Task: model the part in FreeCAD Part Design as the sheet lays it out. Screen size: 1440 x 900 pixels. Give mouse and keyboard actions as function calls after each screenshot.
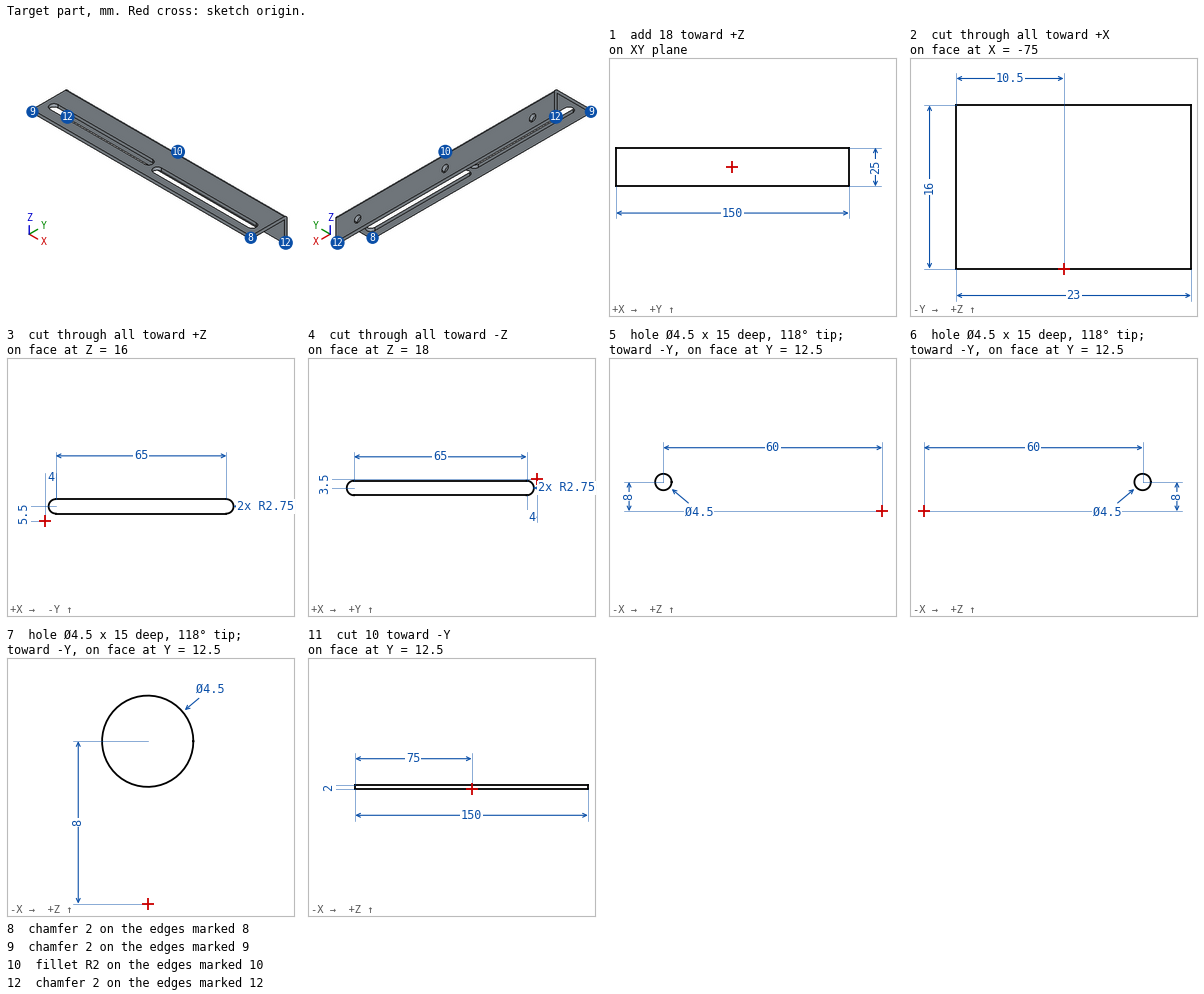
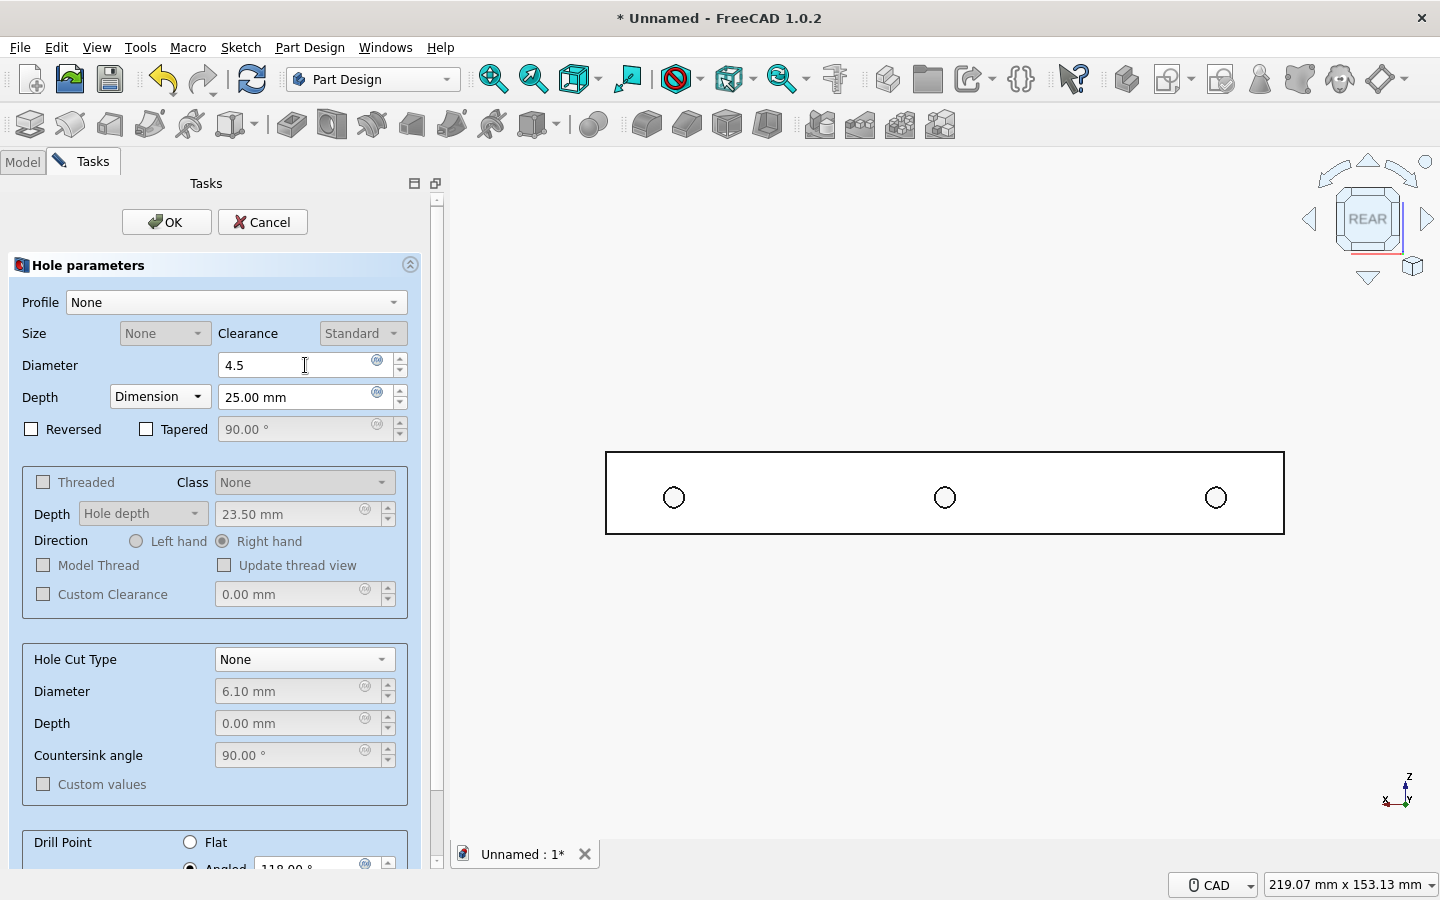
triple_click(305, 397)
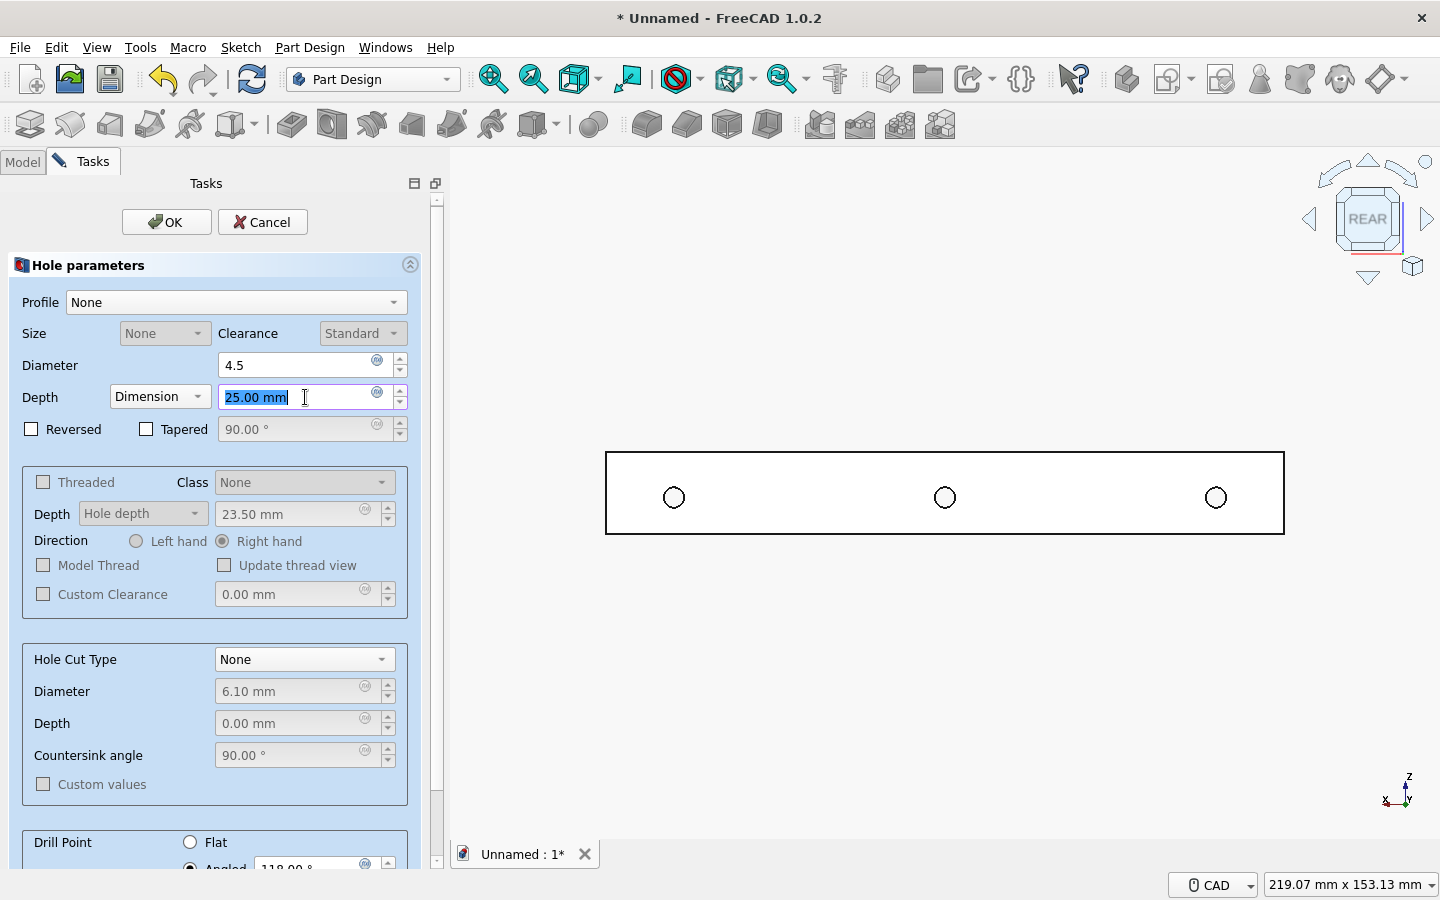
text(15)
key(Tab)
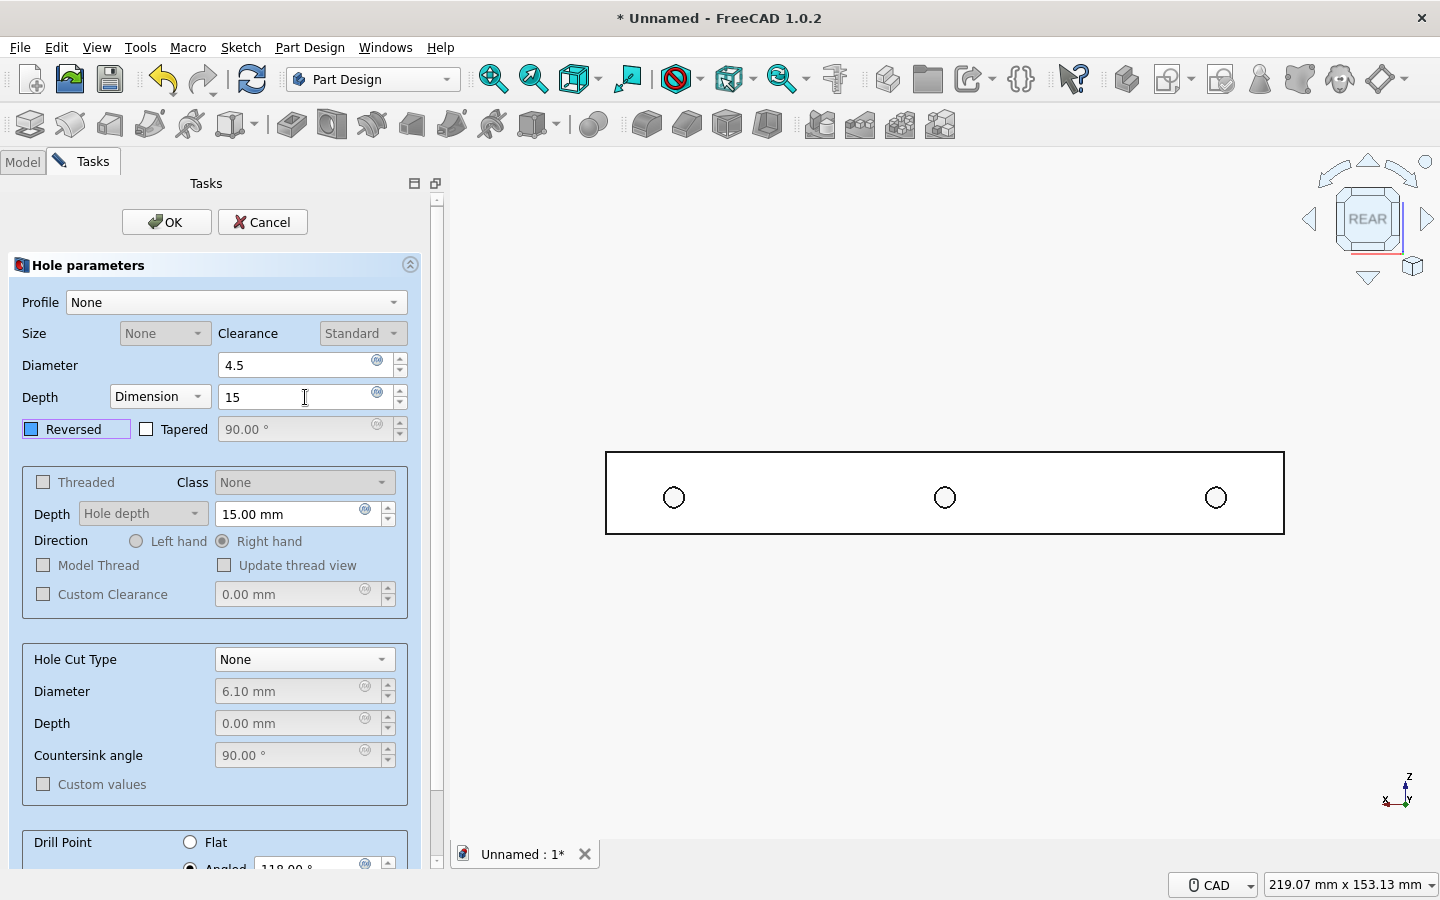
click(167, 222)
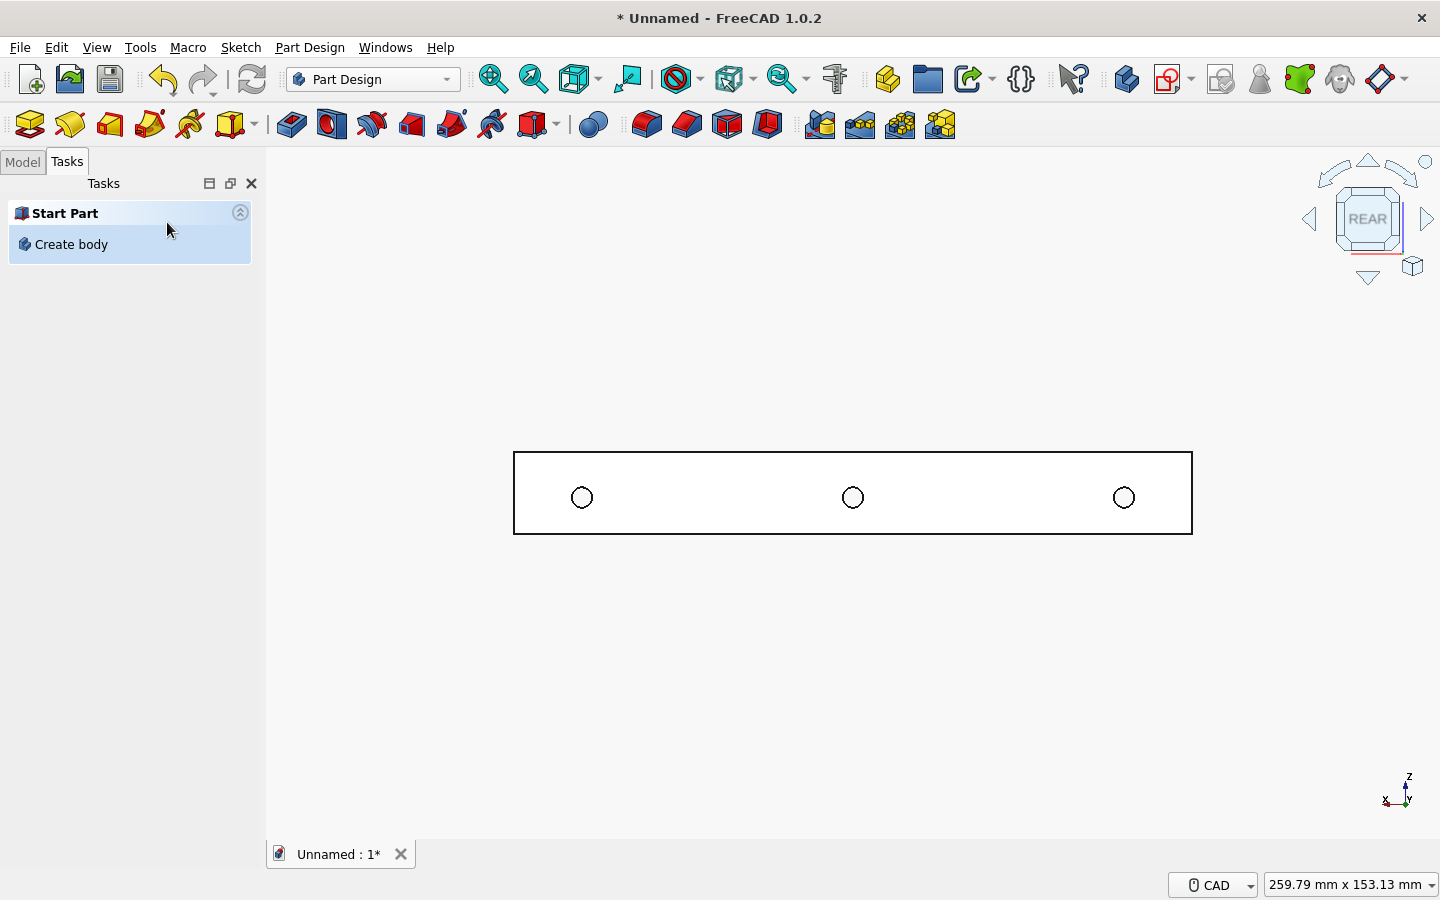
scroll(514, 456, up, 8)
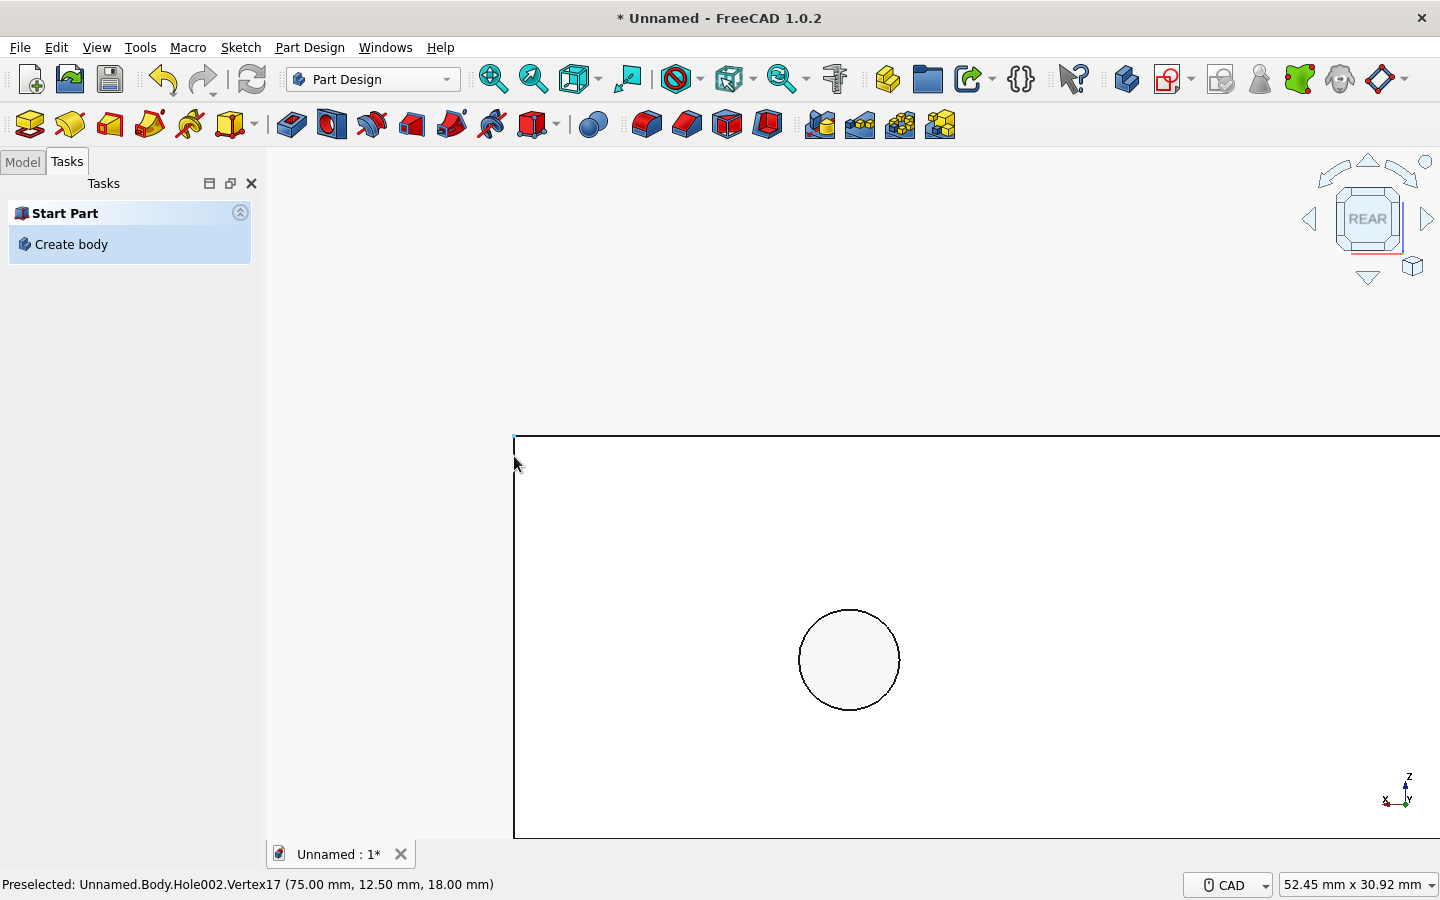
click(494, 80)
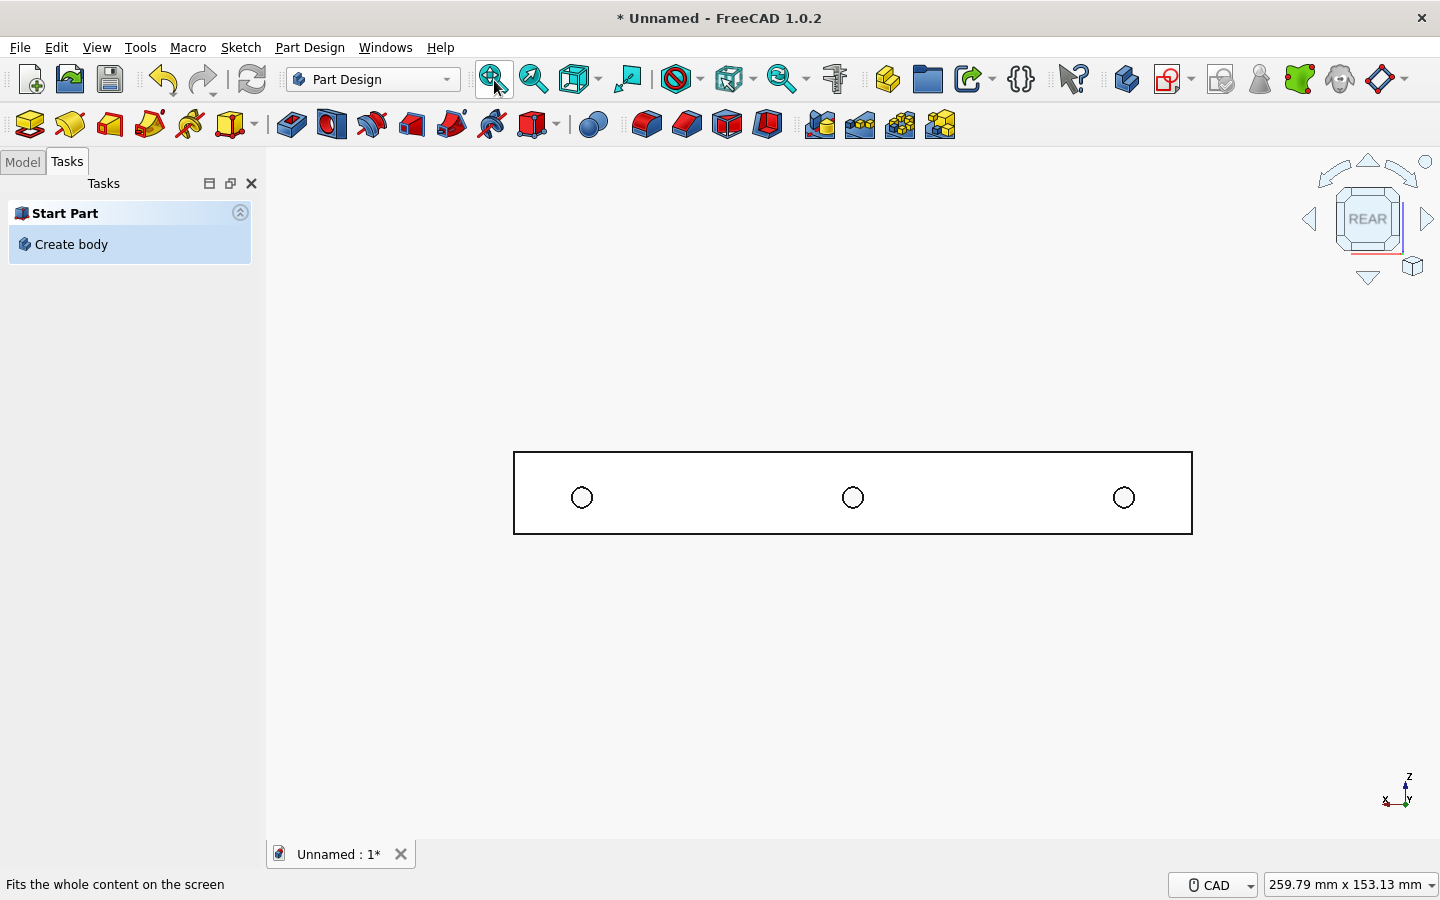
key(0)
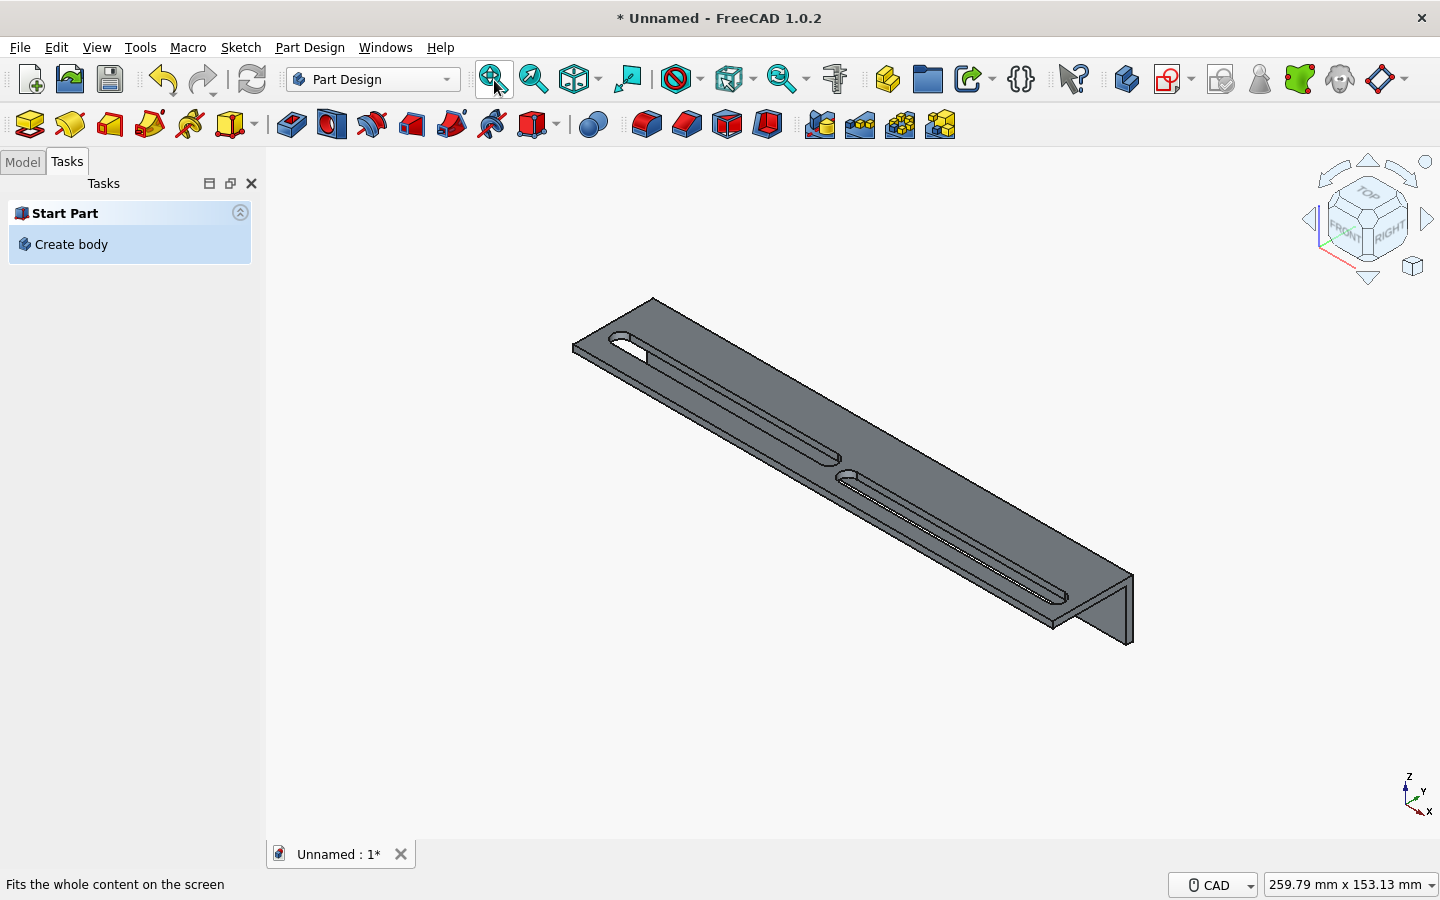
scroll(1053, 624, up, 8)